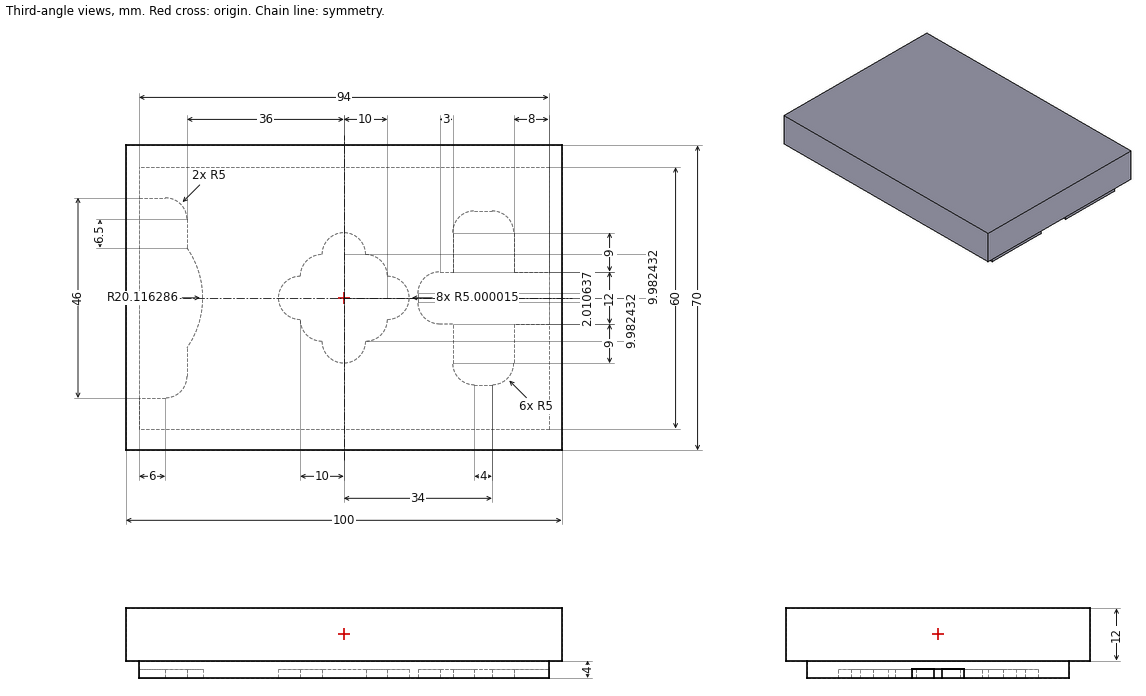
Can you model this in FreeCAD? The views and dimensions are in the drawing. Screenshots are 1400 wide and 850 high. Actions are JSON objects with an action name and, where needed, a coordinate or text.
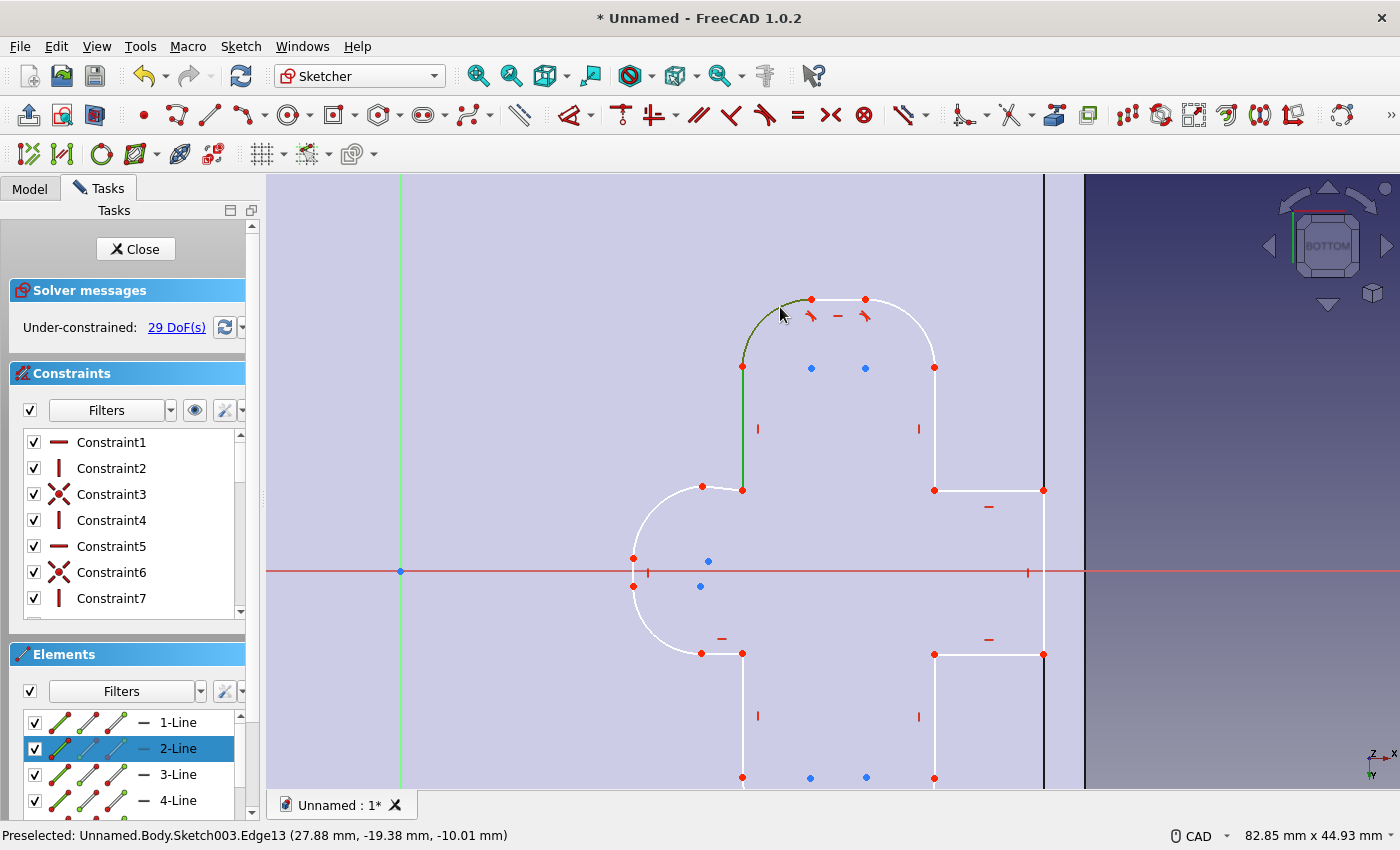
{"action": "left_click", "coordinate": [765, 116]}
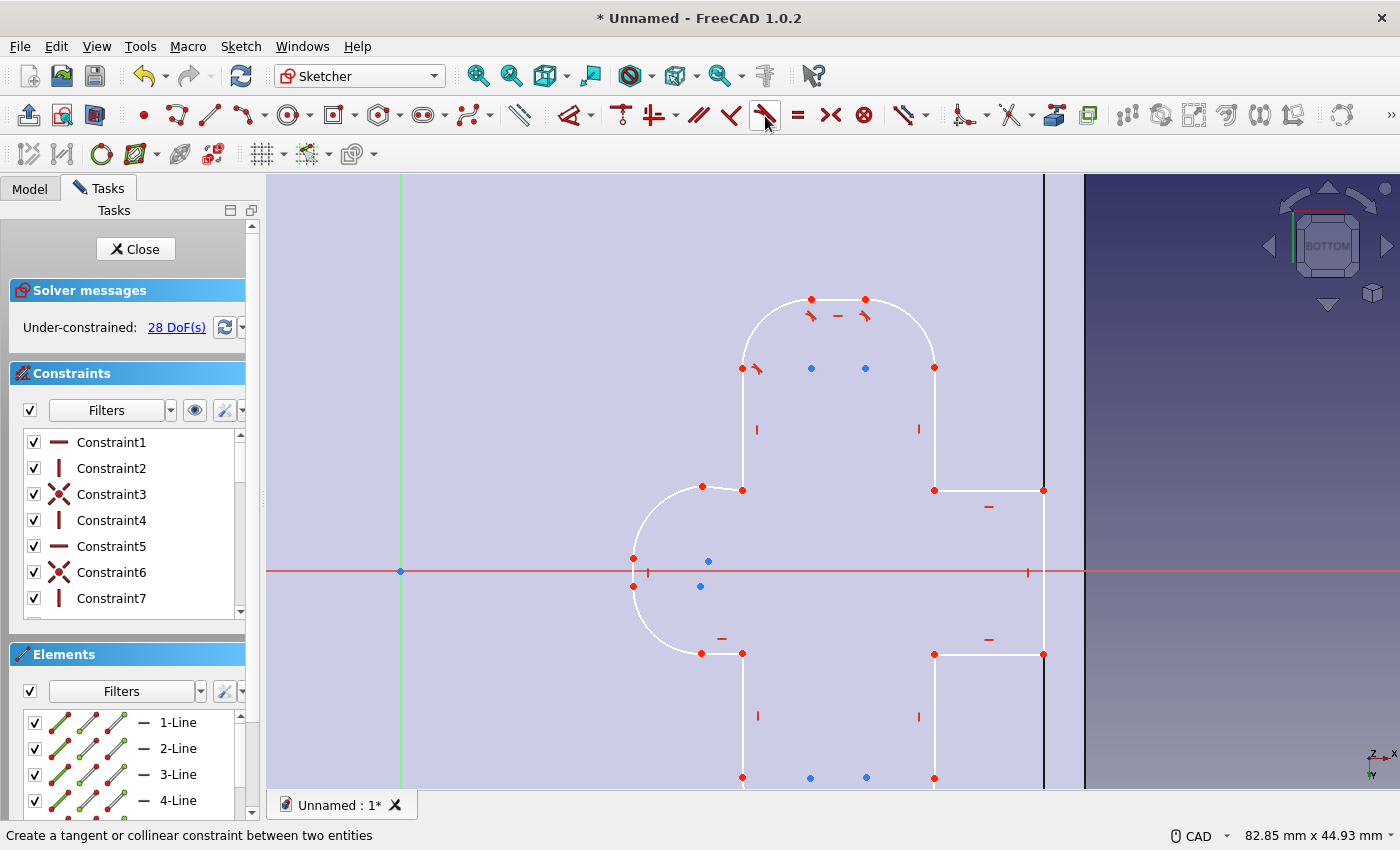
{"action": "left_click", "coordinate": [731, 489]}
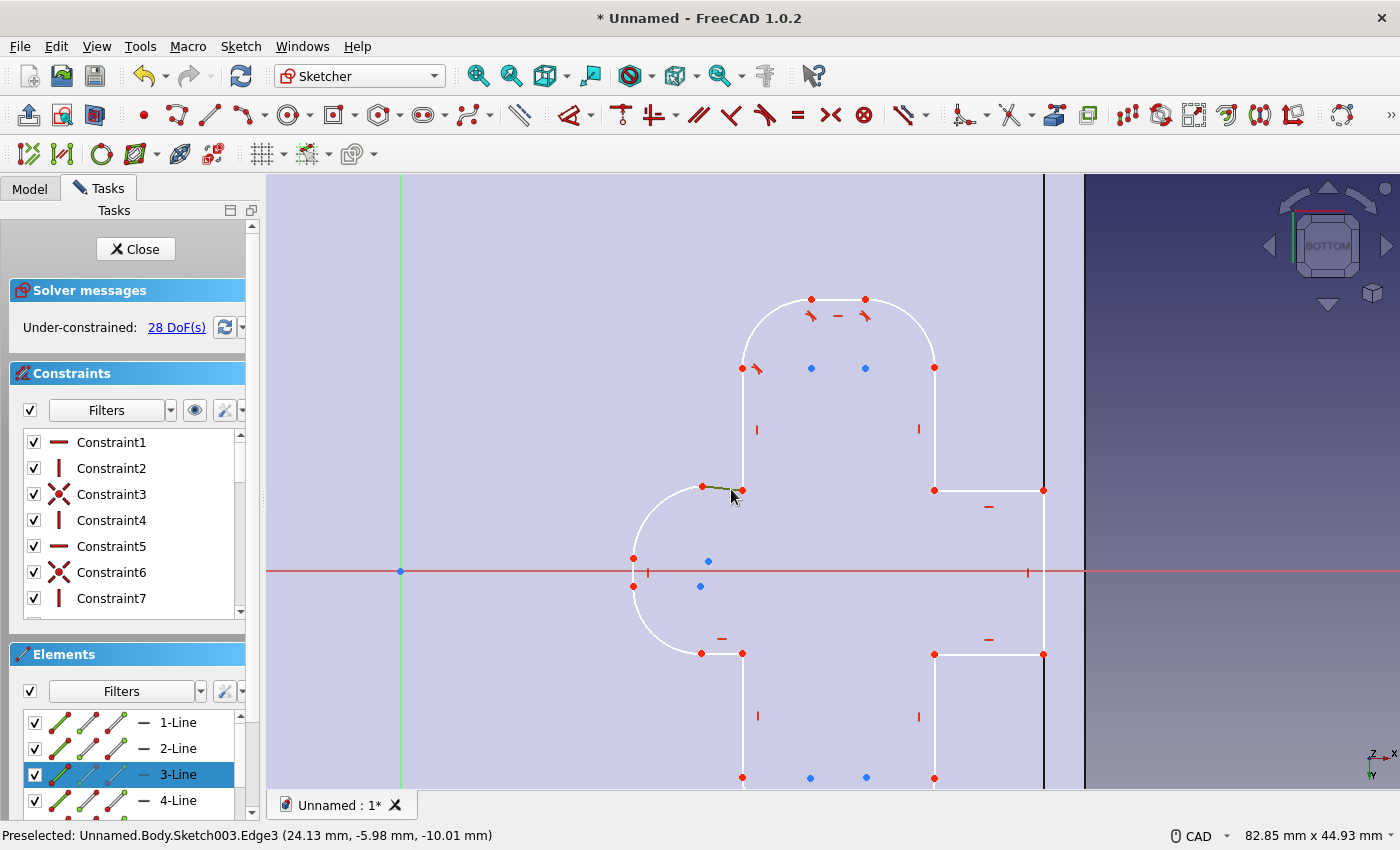
{"action": "left_click", "coordinate": [671, 496]}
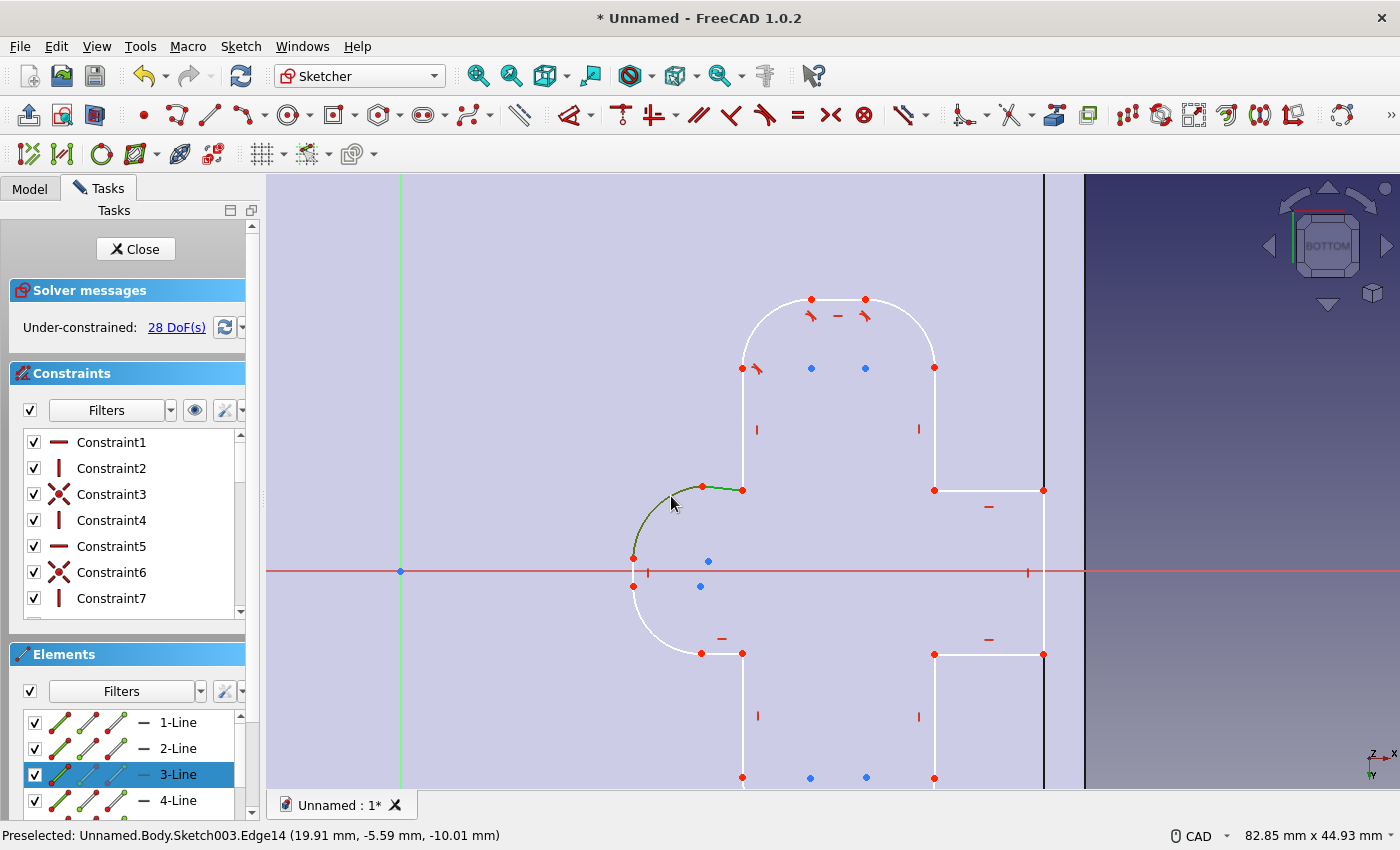
{"action": "left_click", "coordinate": [765, 116]}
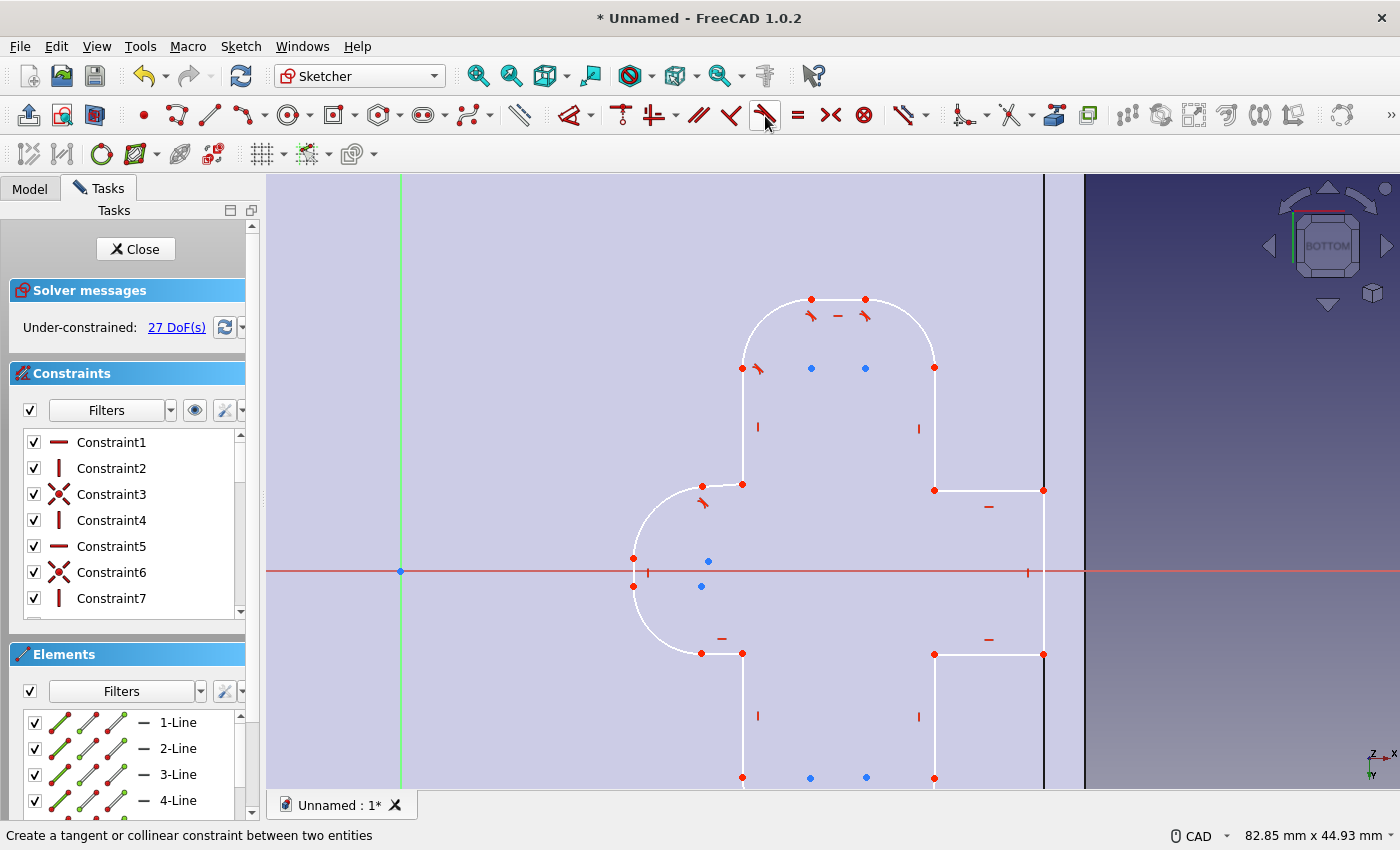
{"action": "scroll", "coordinate": [634, 569], "scroll_direction": "up", "scroll_amount": 2}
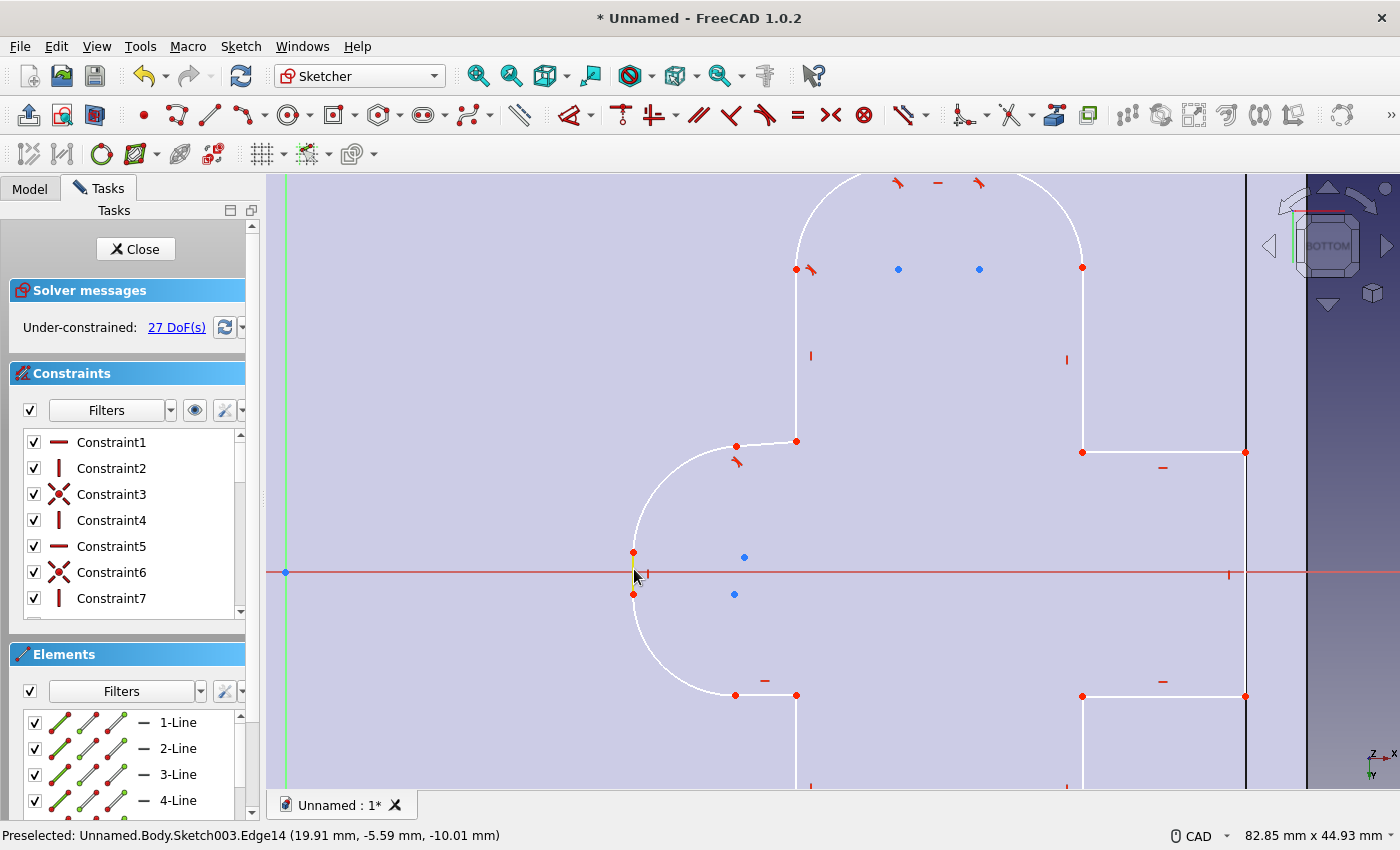
{"action": "left_click", "coordinate": [633, 569]}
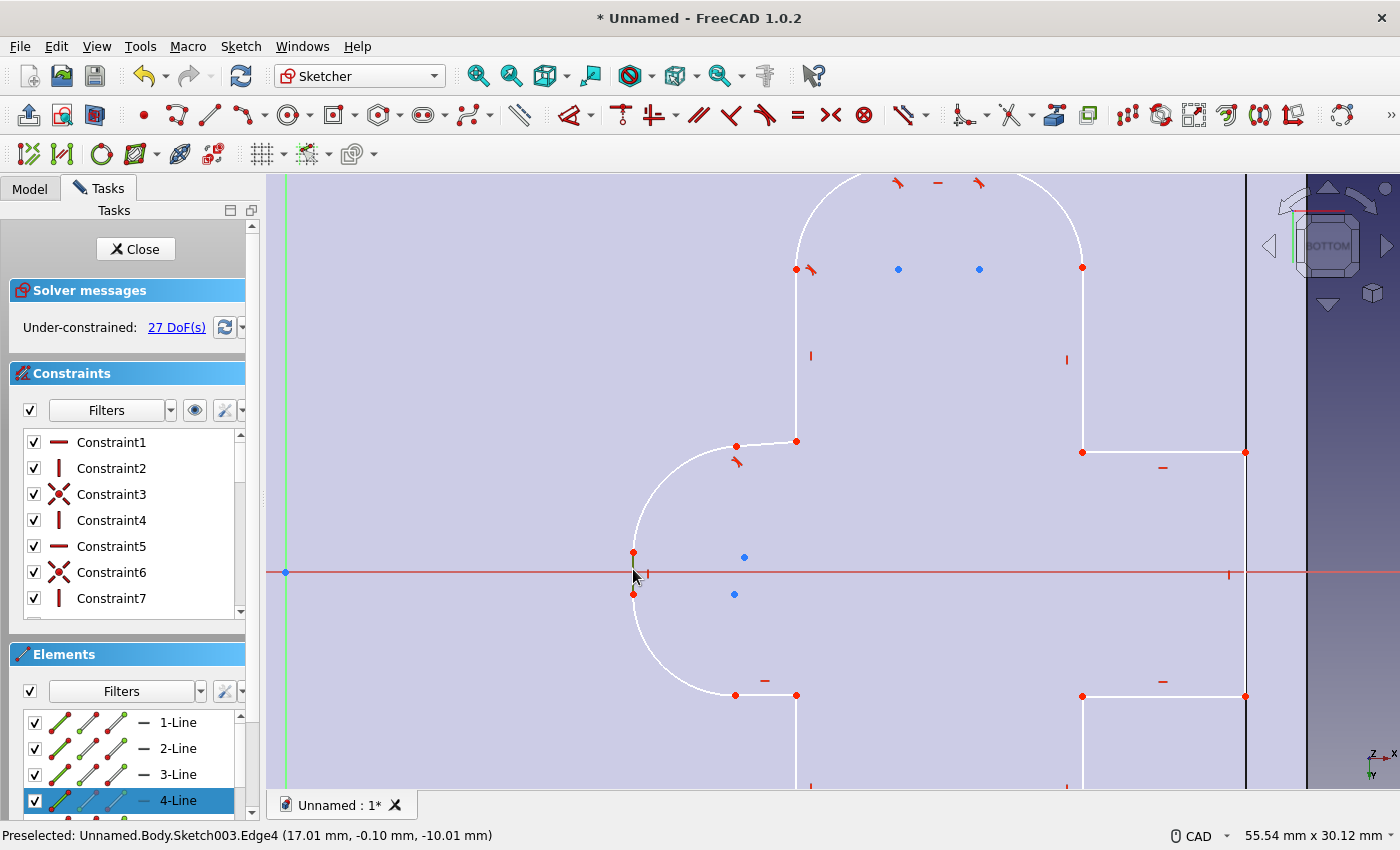
{"action": "left_click", "coordinate": [690, 460]}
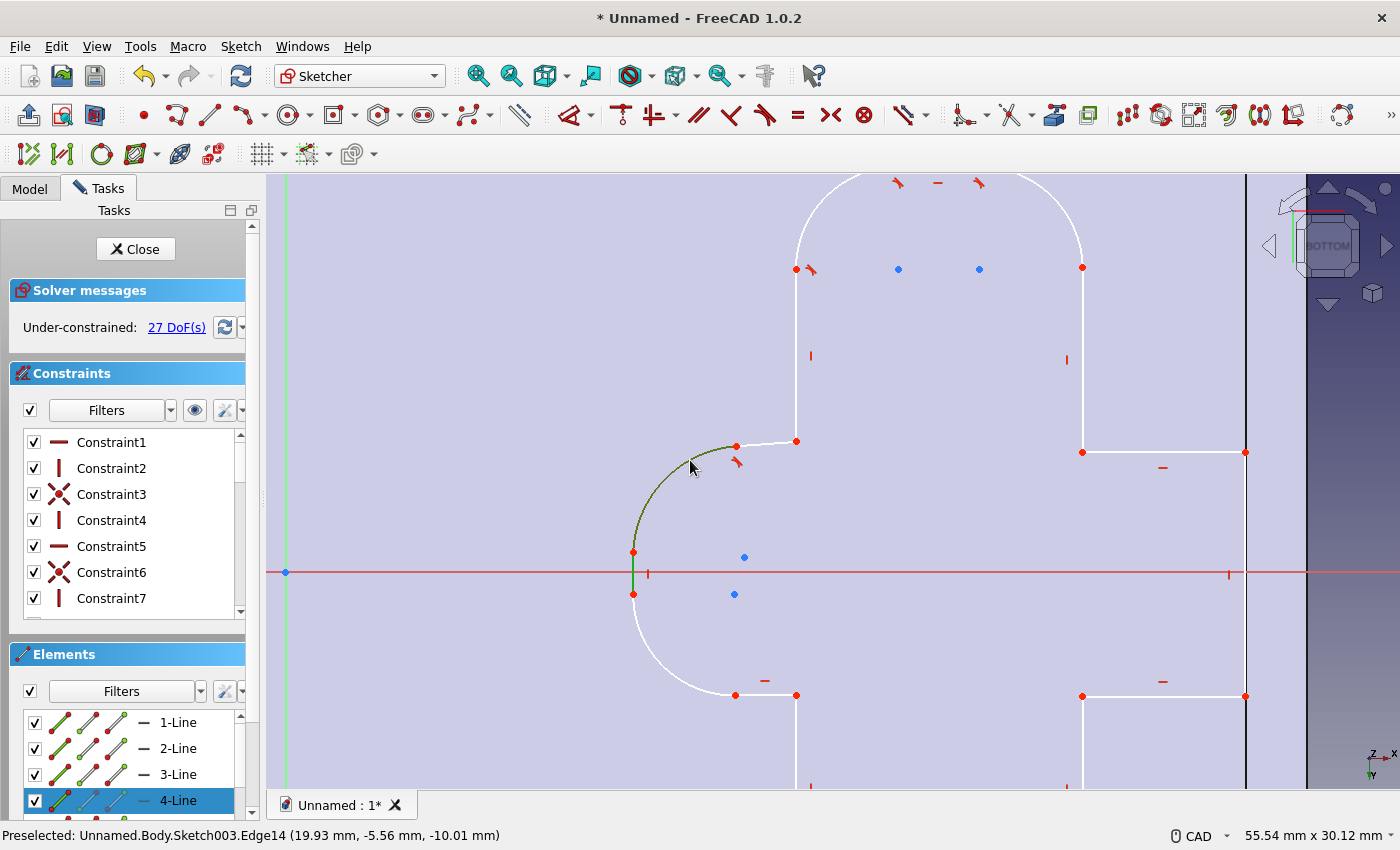
{"action": "left_click", "coordinate": [765, 116]}